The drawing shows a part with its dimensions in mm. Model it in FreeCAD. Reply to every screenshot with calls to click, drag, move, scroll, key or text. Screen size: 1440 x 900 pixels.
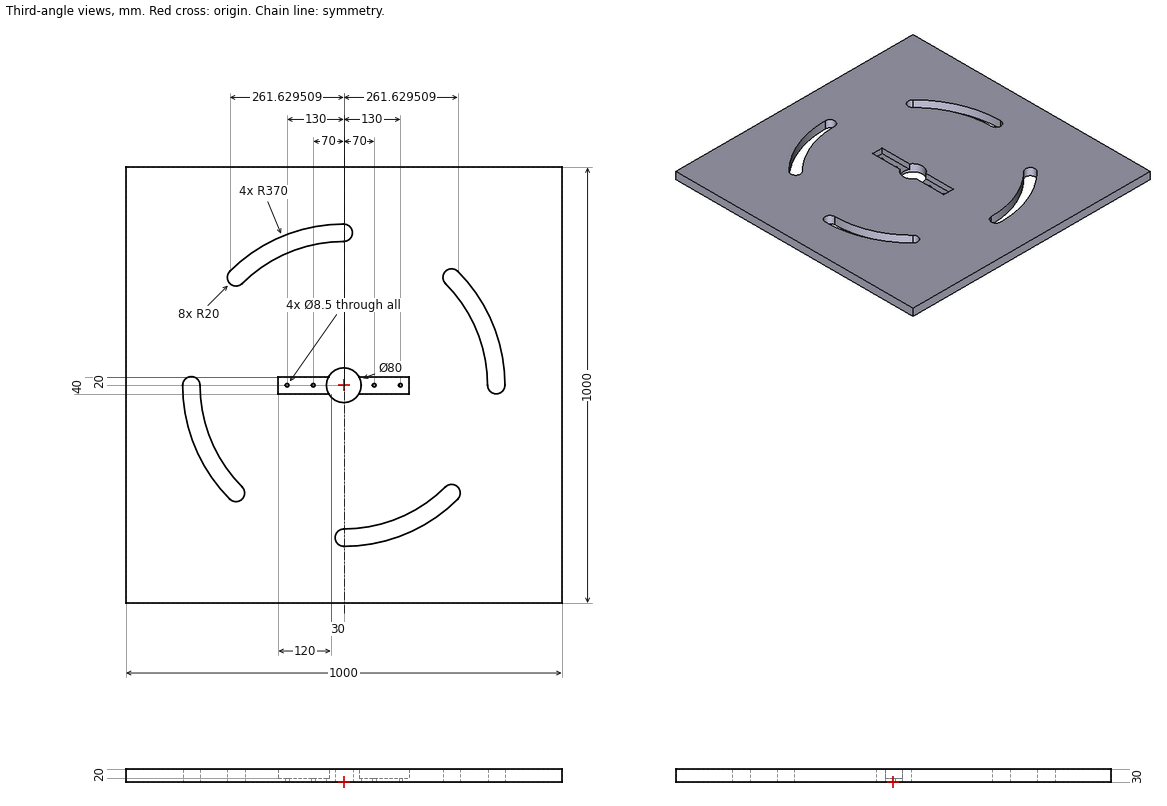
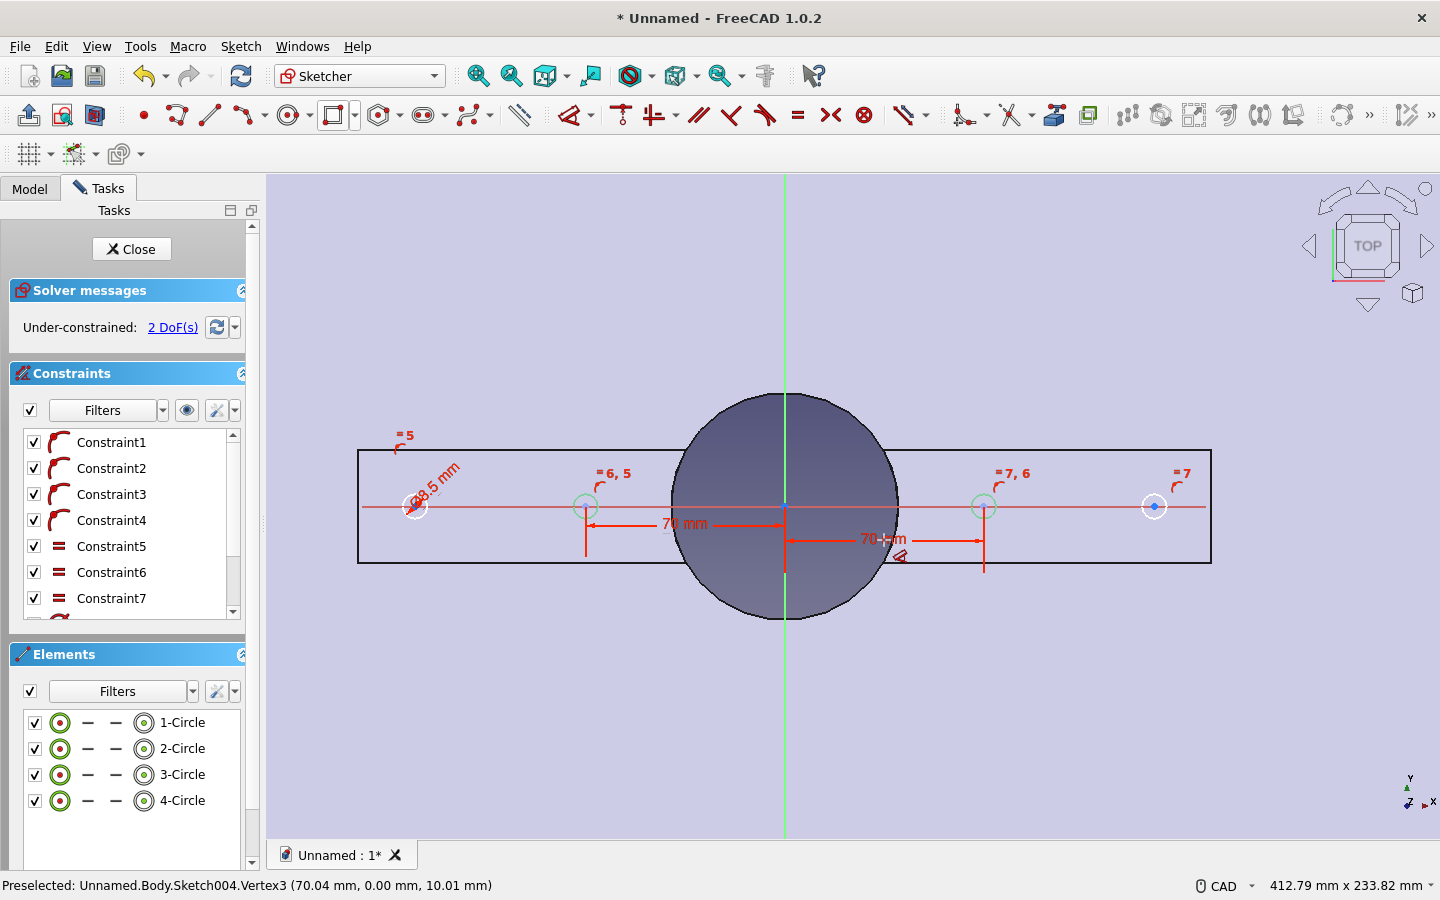
click(415, 506)
click(600, 540)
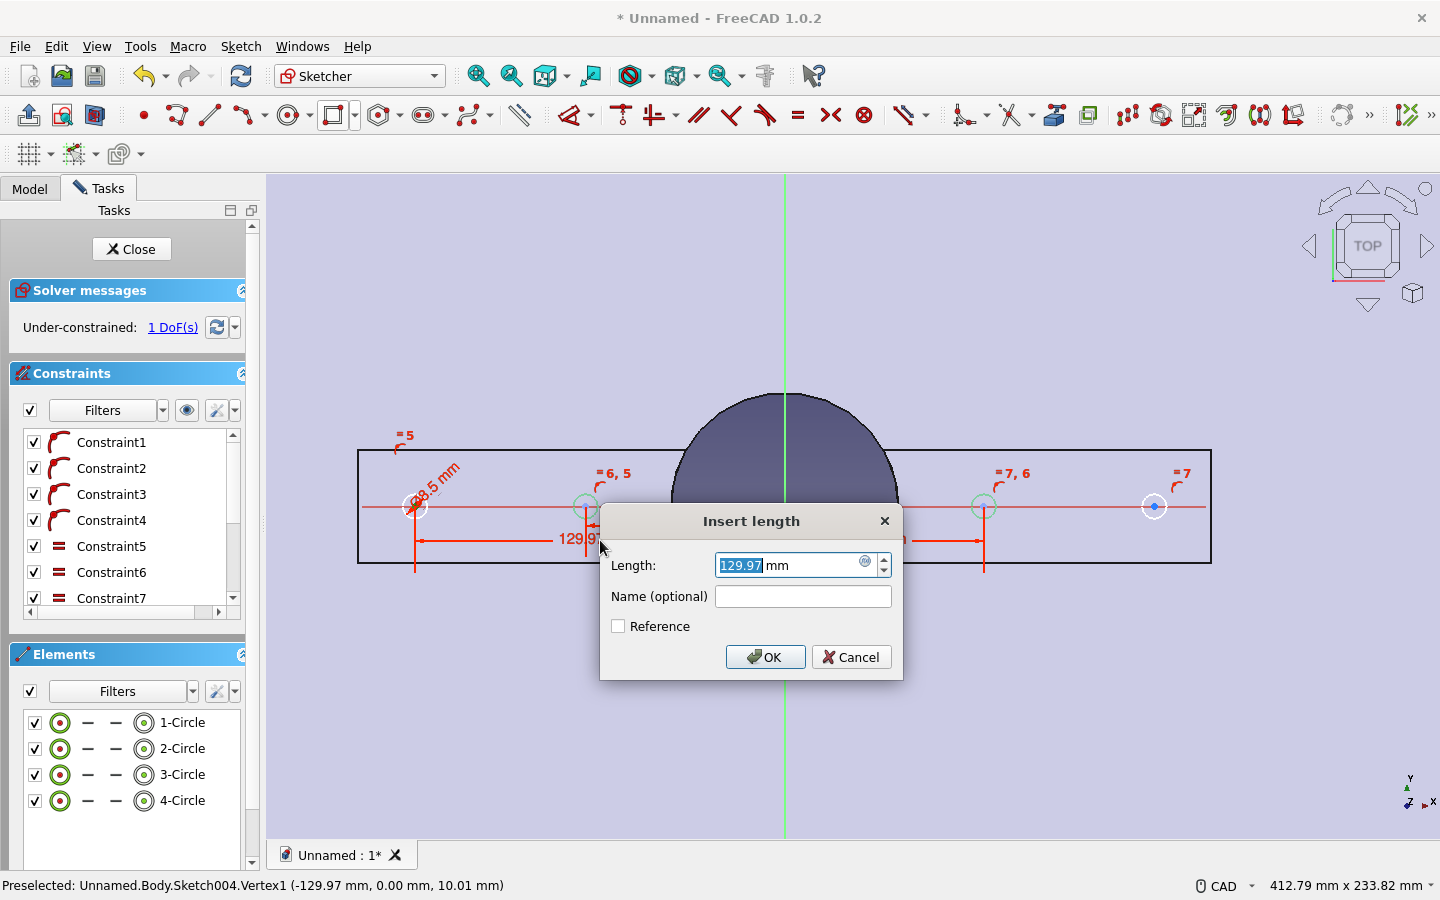
text(130)
key(Return)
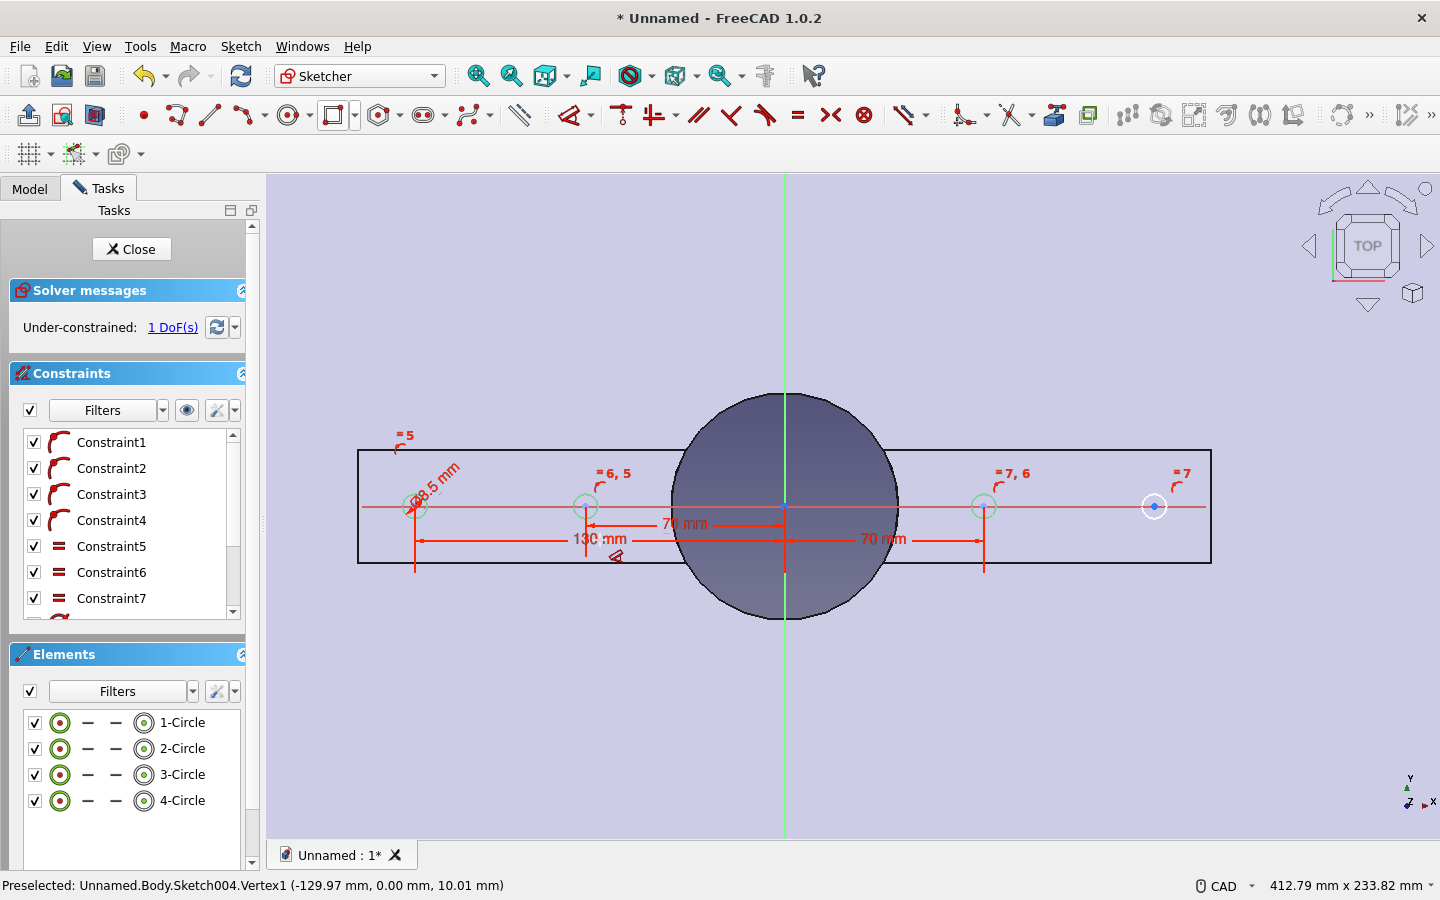
click(1154, 506)
click(970, 540)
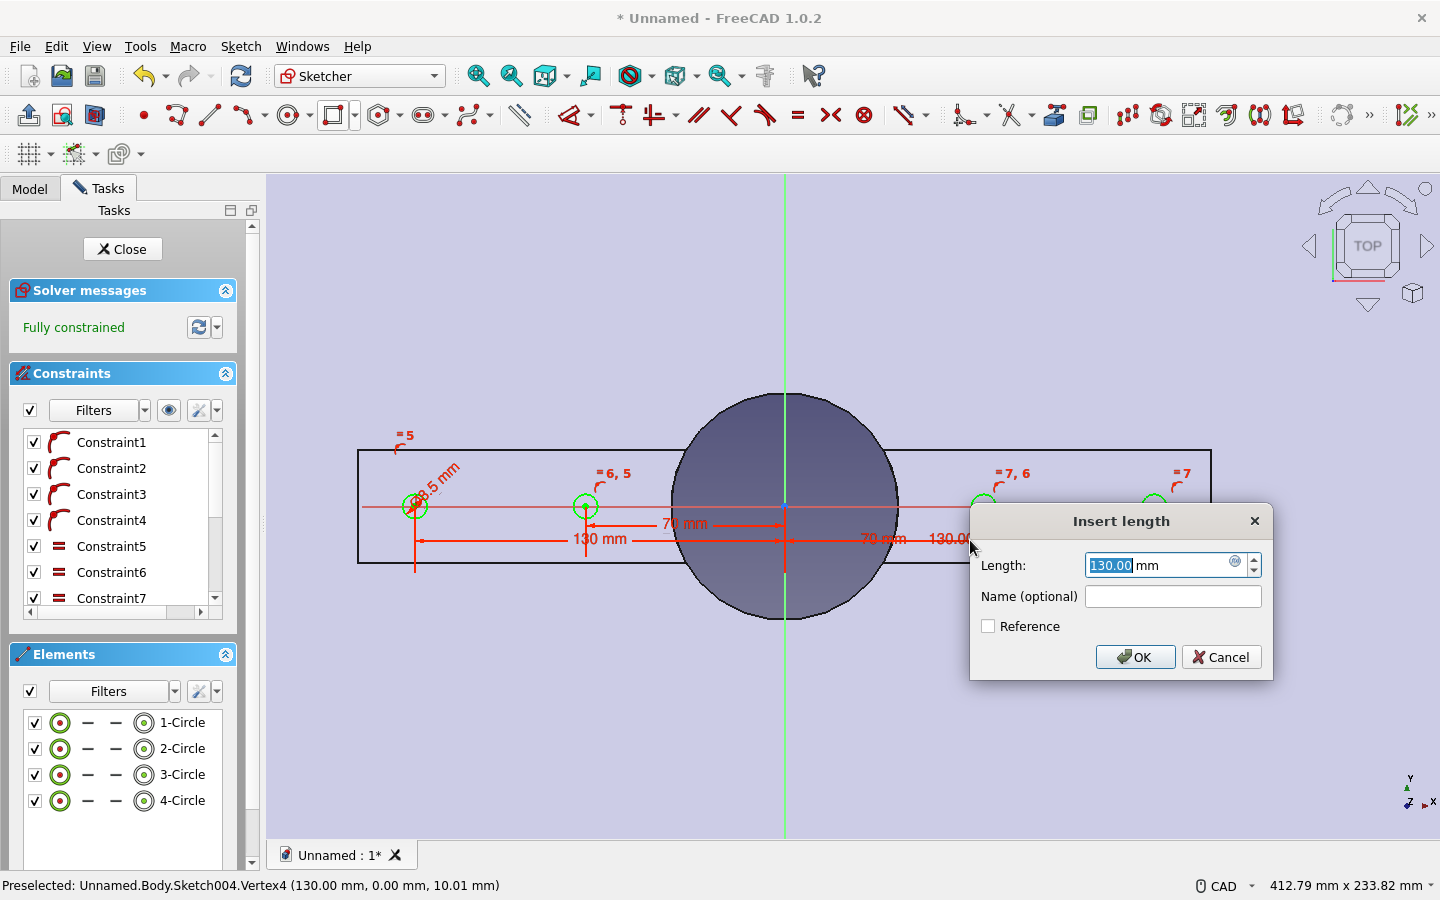
text(130)
key(Return)
key(Escape)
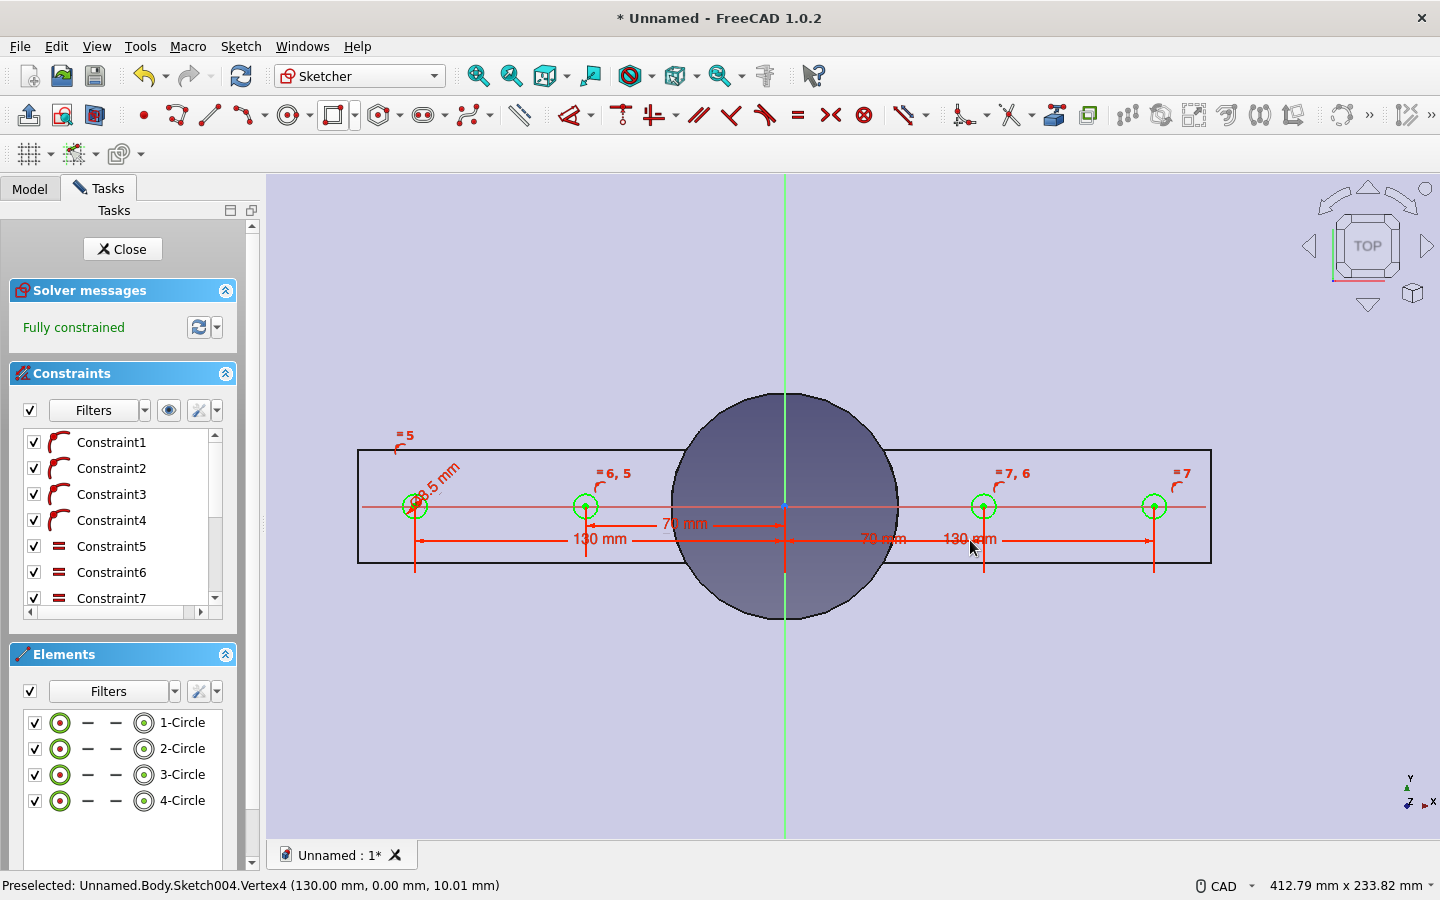
click(123, 249)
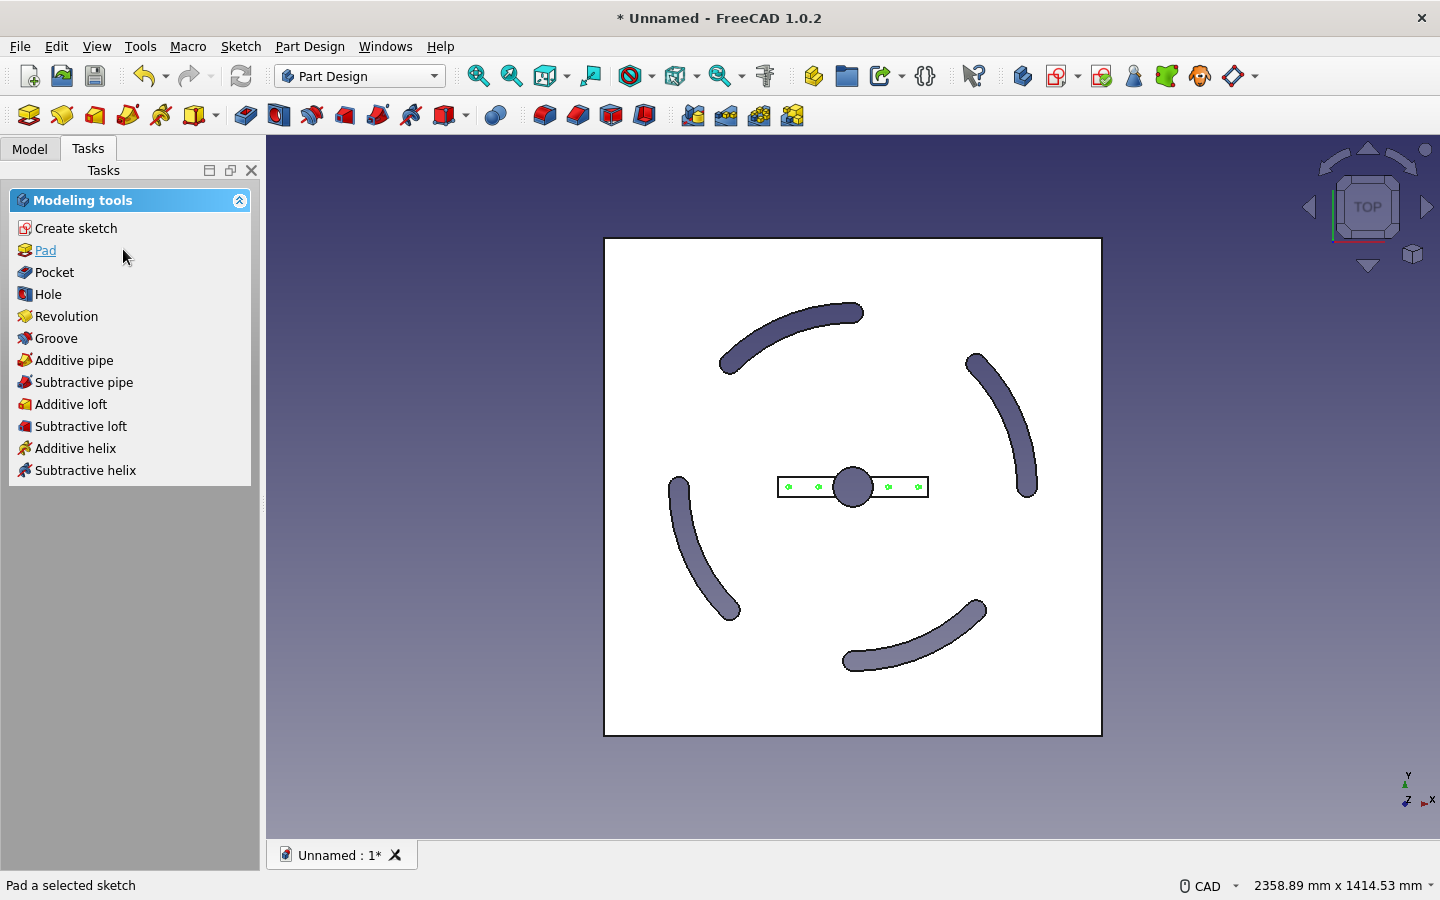
click(279, 116)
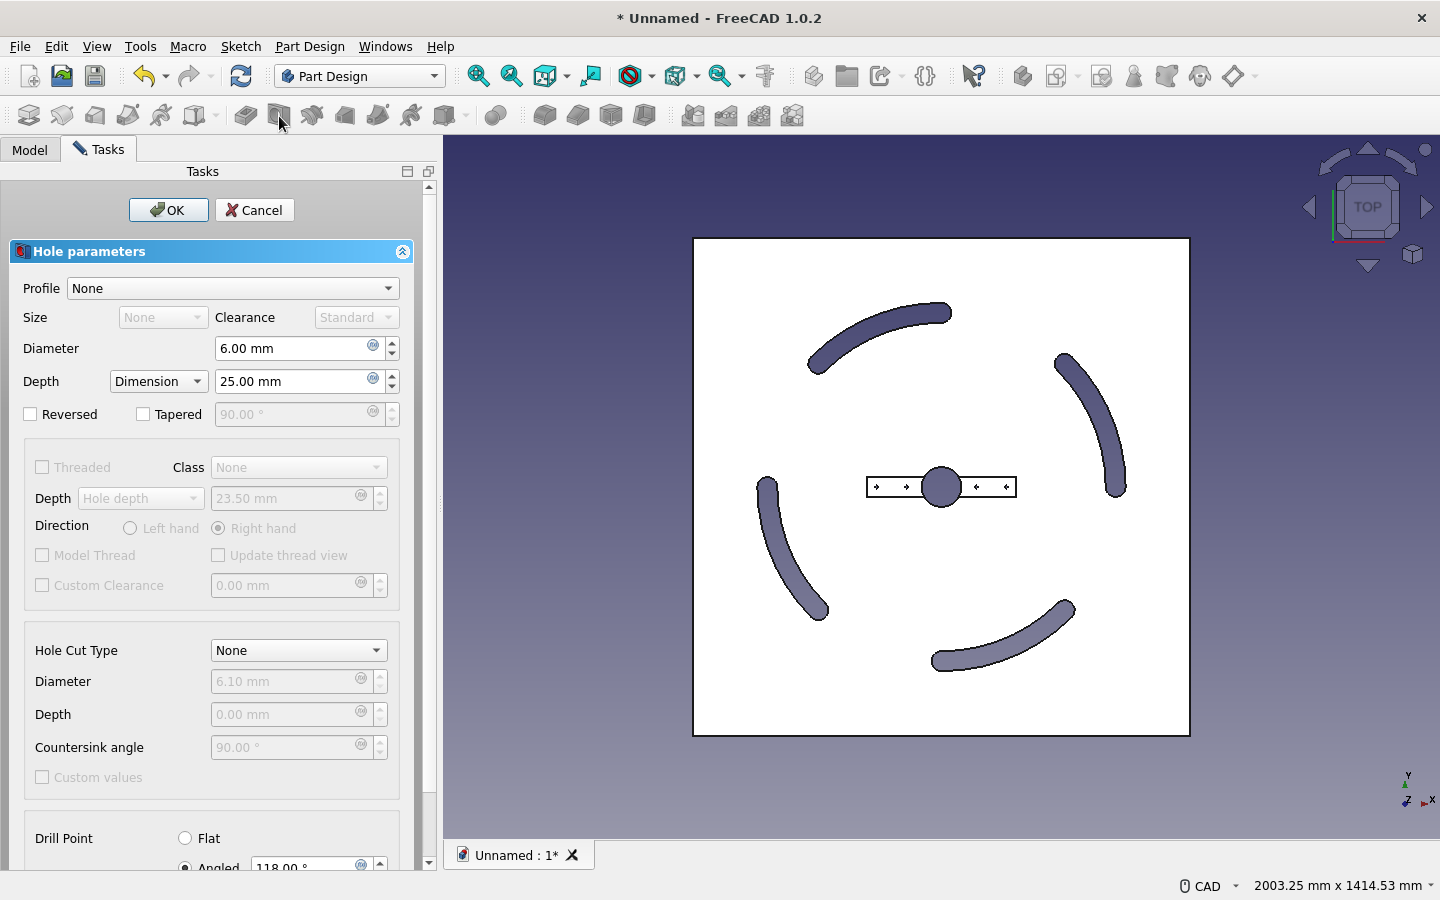
triple_click(300, 348)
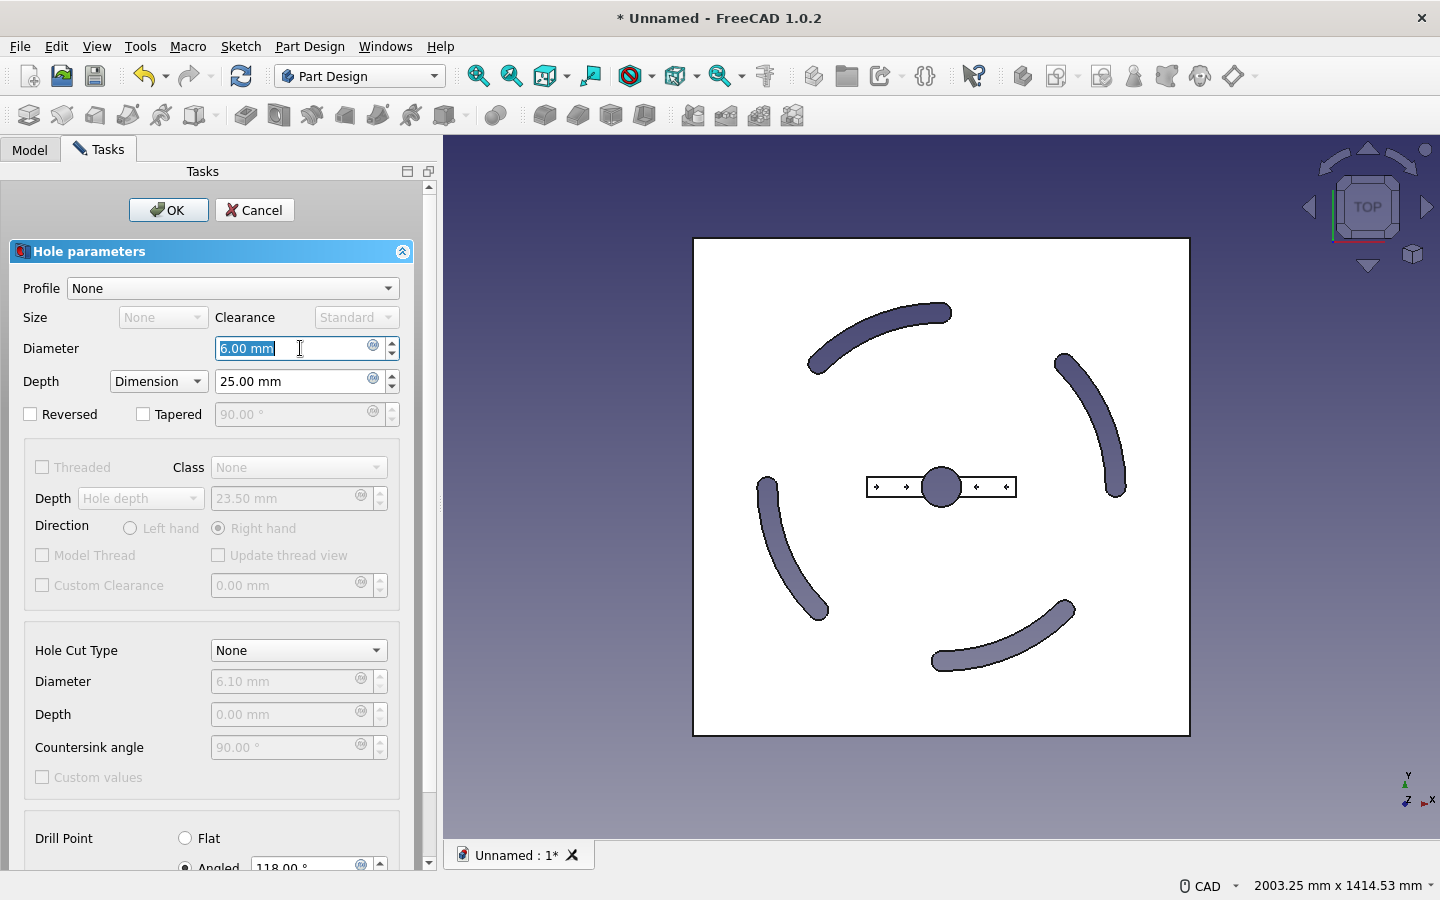
text(8.5)
key(Tab)